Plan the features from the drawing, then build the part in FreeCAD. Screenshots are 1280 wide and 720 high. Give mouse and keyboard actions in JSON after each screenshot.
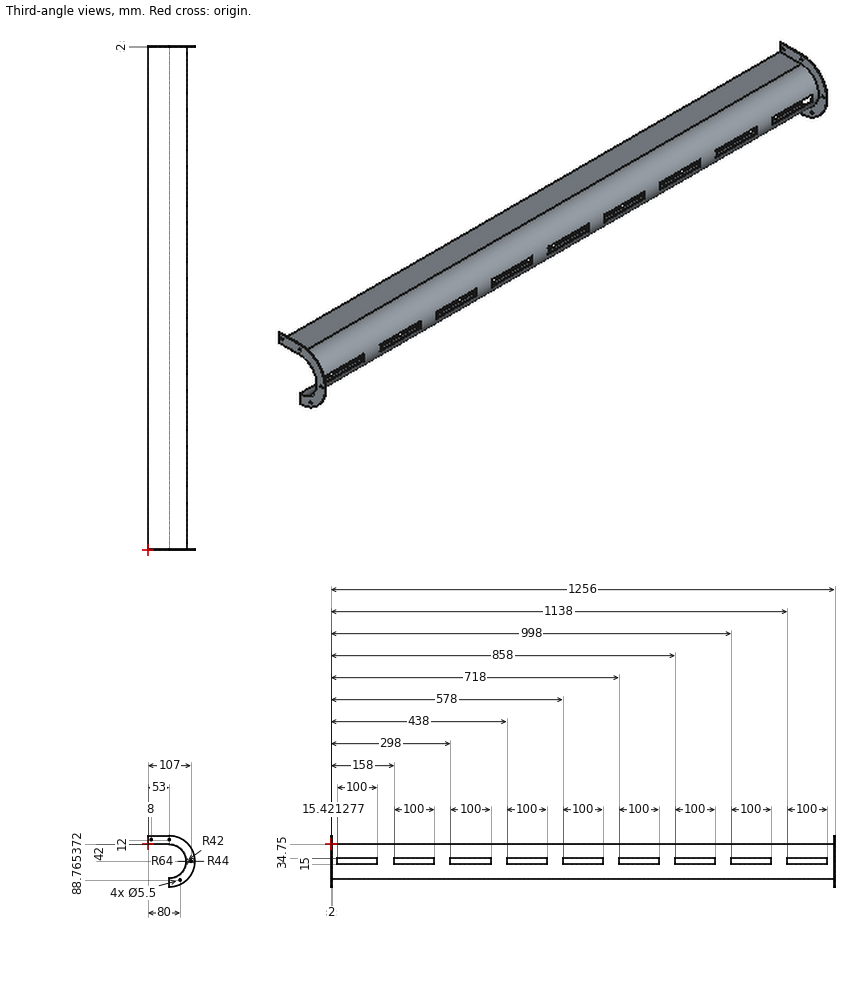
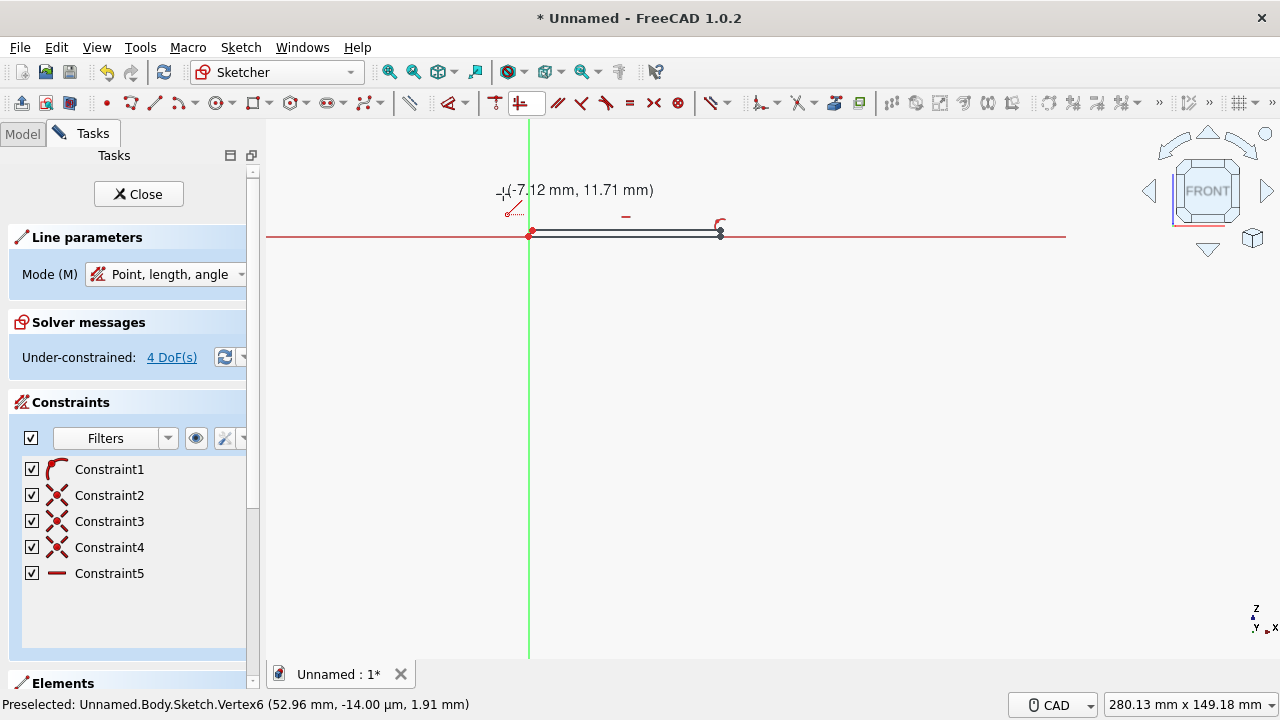
{"action": "left_click", "coordinate": [721, 548]}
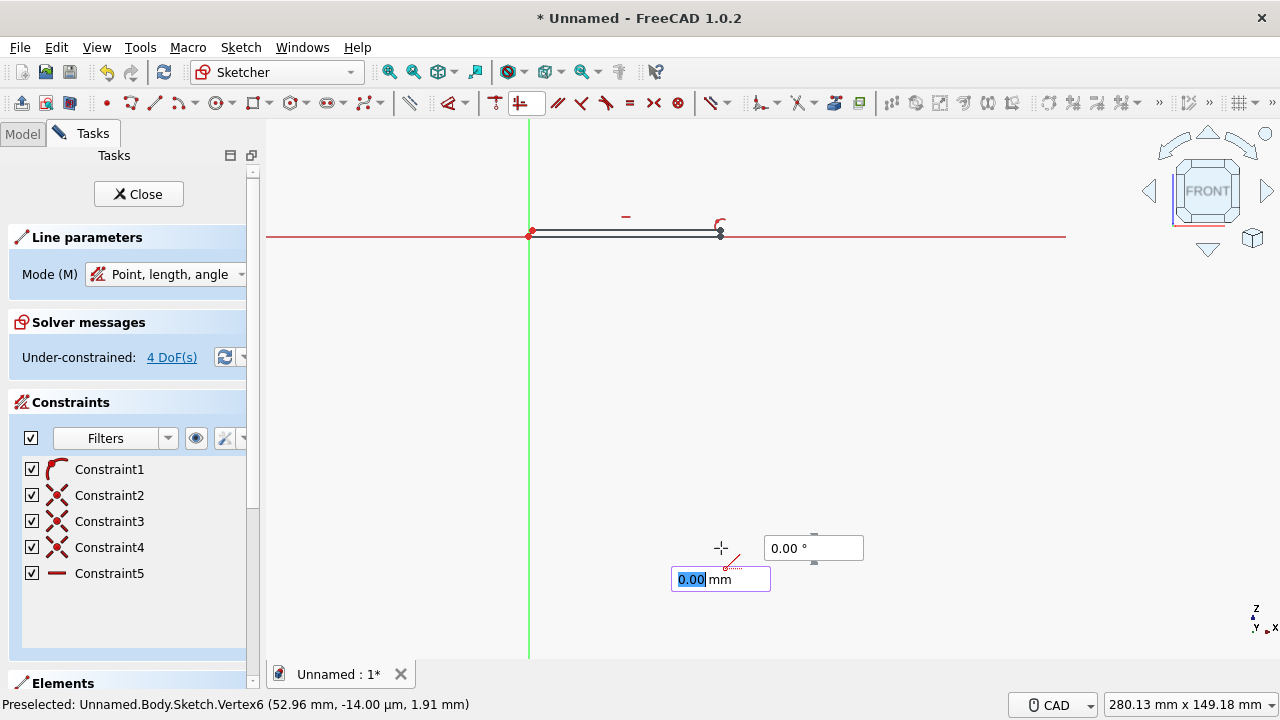
{"action": "scroll", "coordinate": [721, 541], "scroll_direction": "up", "scroll_amount": 4}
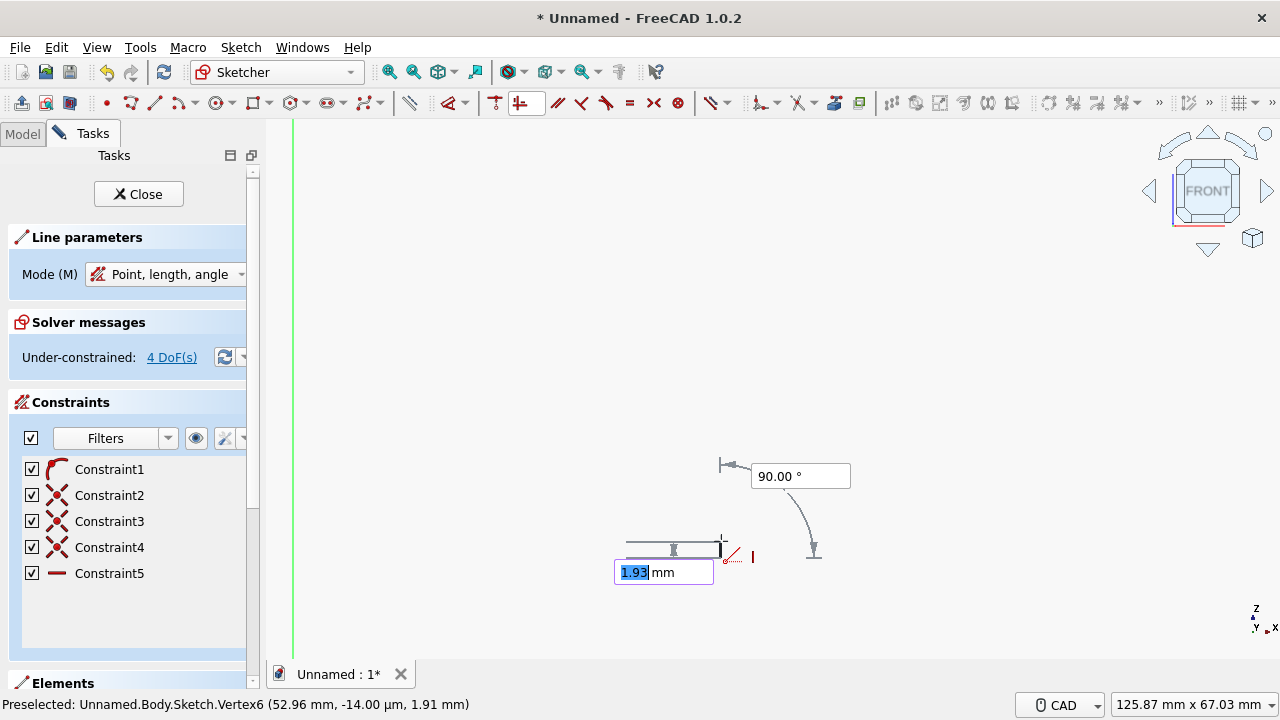
{"action": "left_click", "coordinate": [720, 540]}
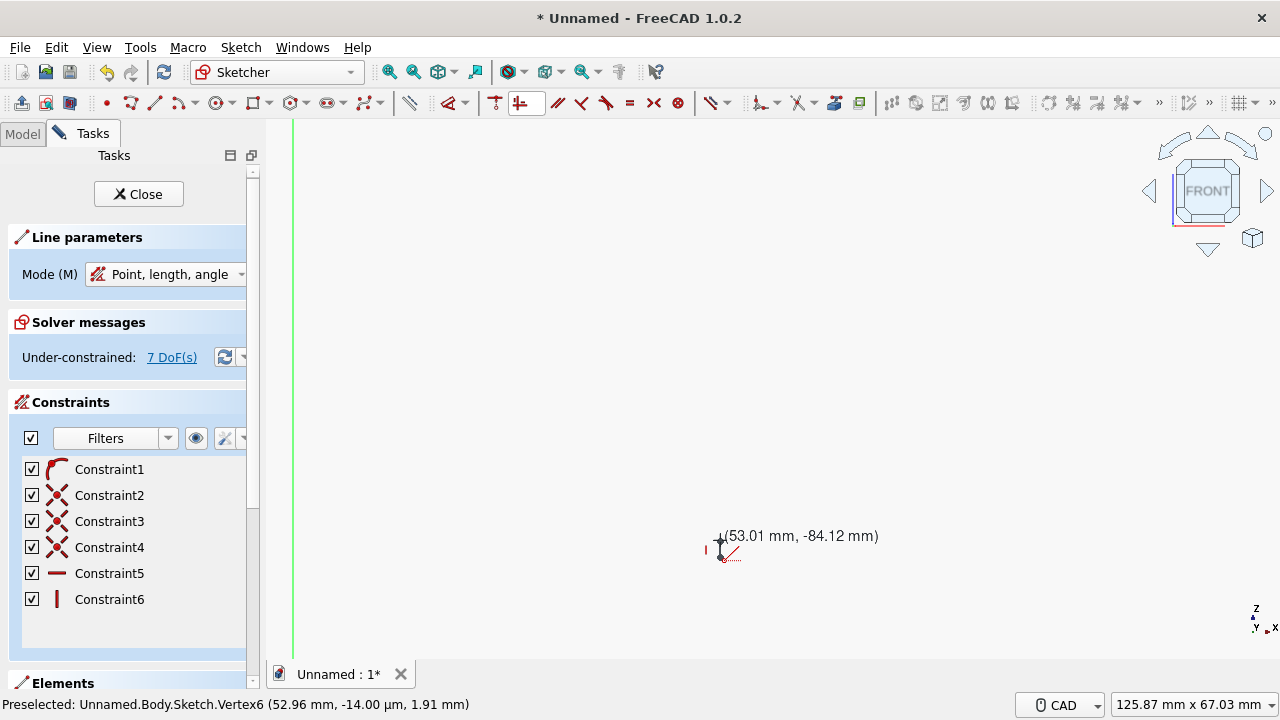
{"action": "left_click", "coordinate": [198, 104]}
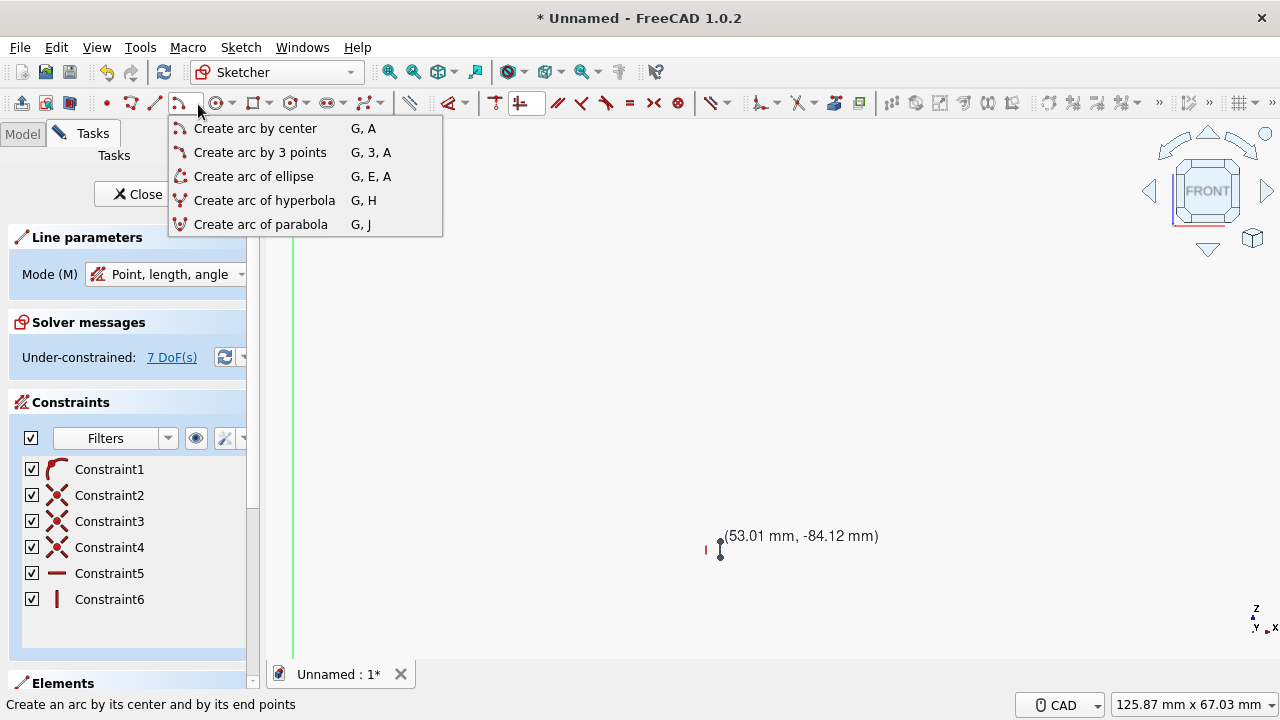
{"action": "left_click", "coordinate": [306, 152]}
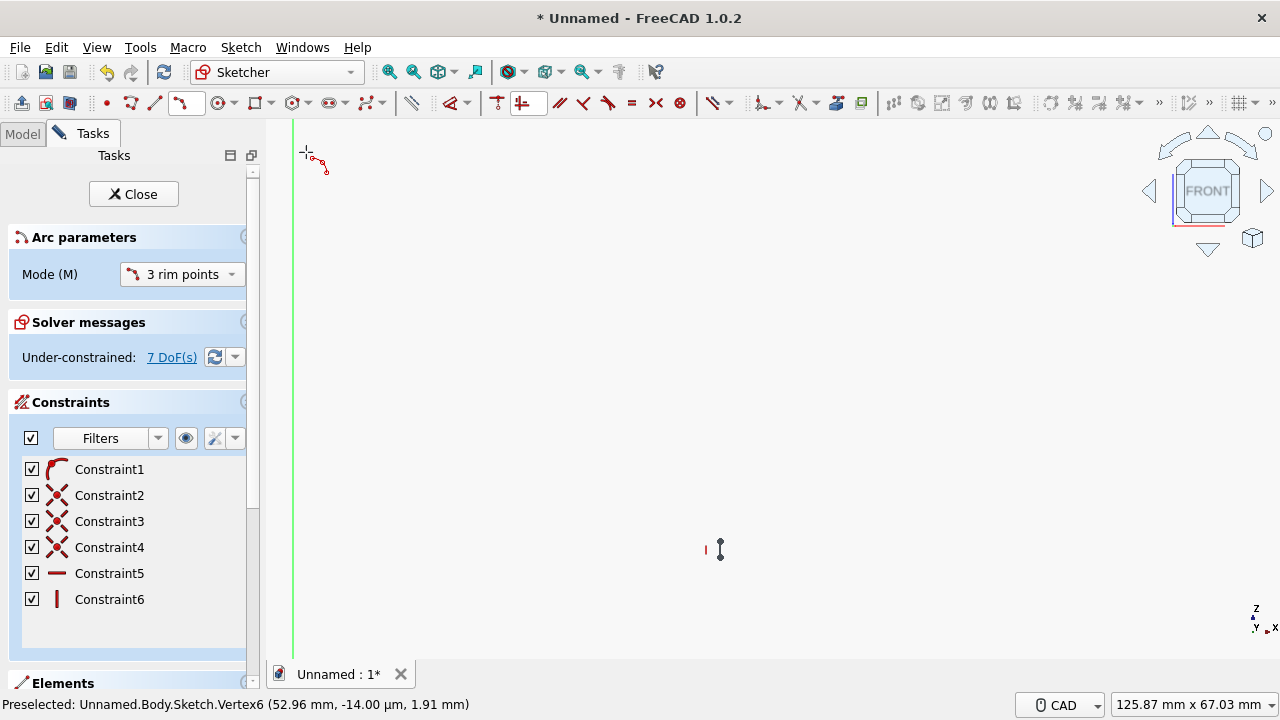
{"action": "scroll", "coordinate": [722, 542], "scroll_direction": "down", "scroll_amount": 4}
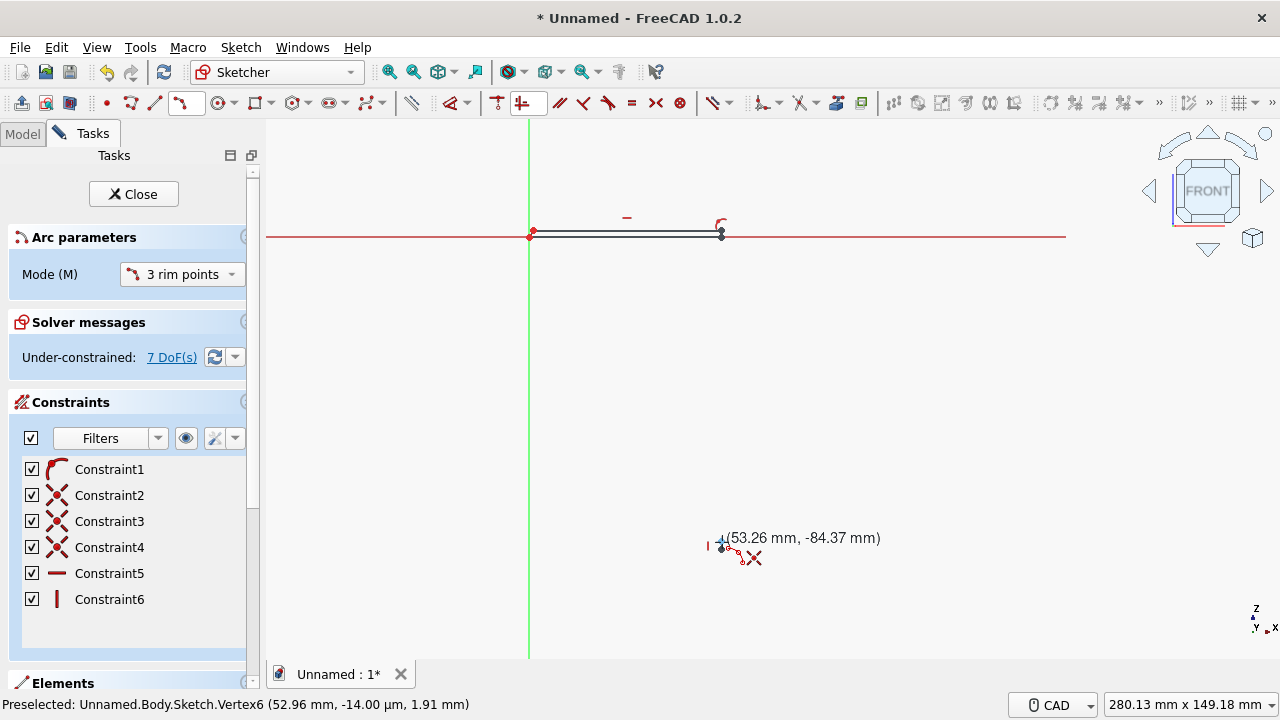
{"action": "scroll", "coordinate": [721, 230], "scroll_direction": "up", "scroll_amount": 4}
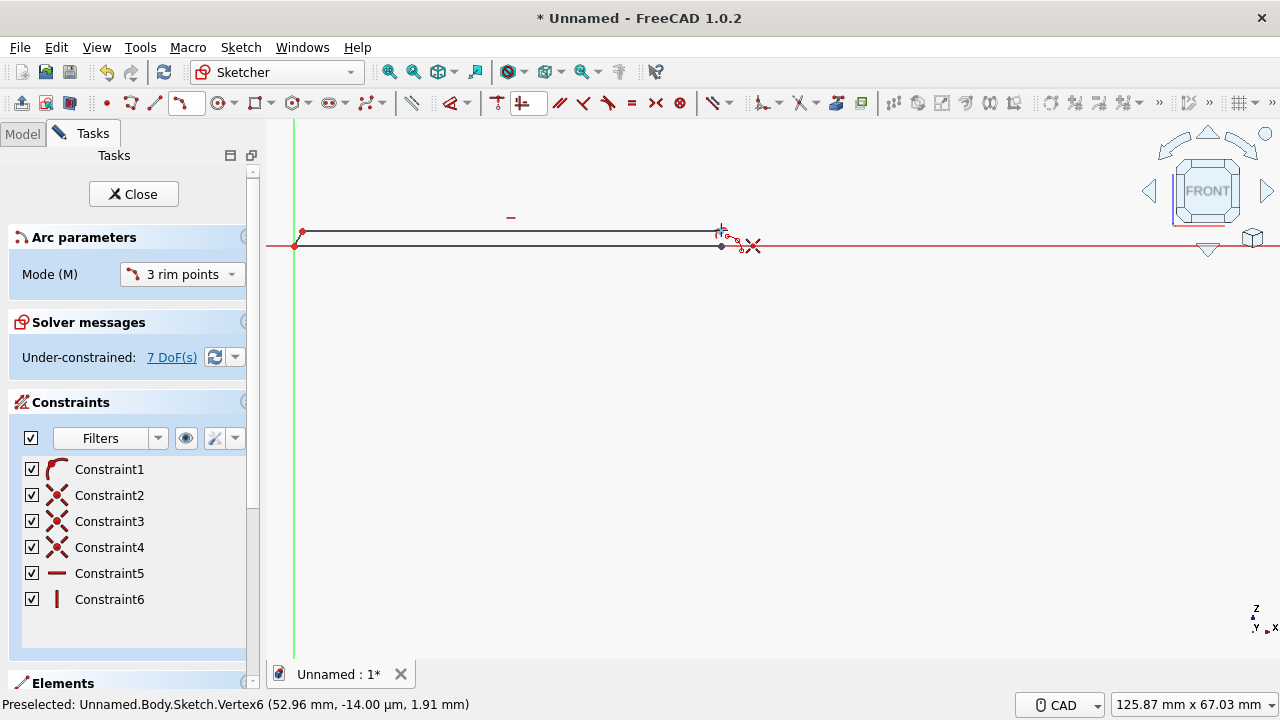
{"action": "left_click", "coordinate": [721, 231]}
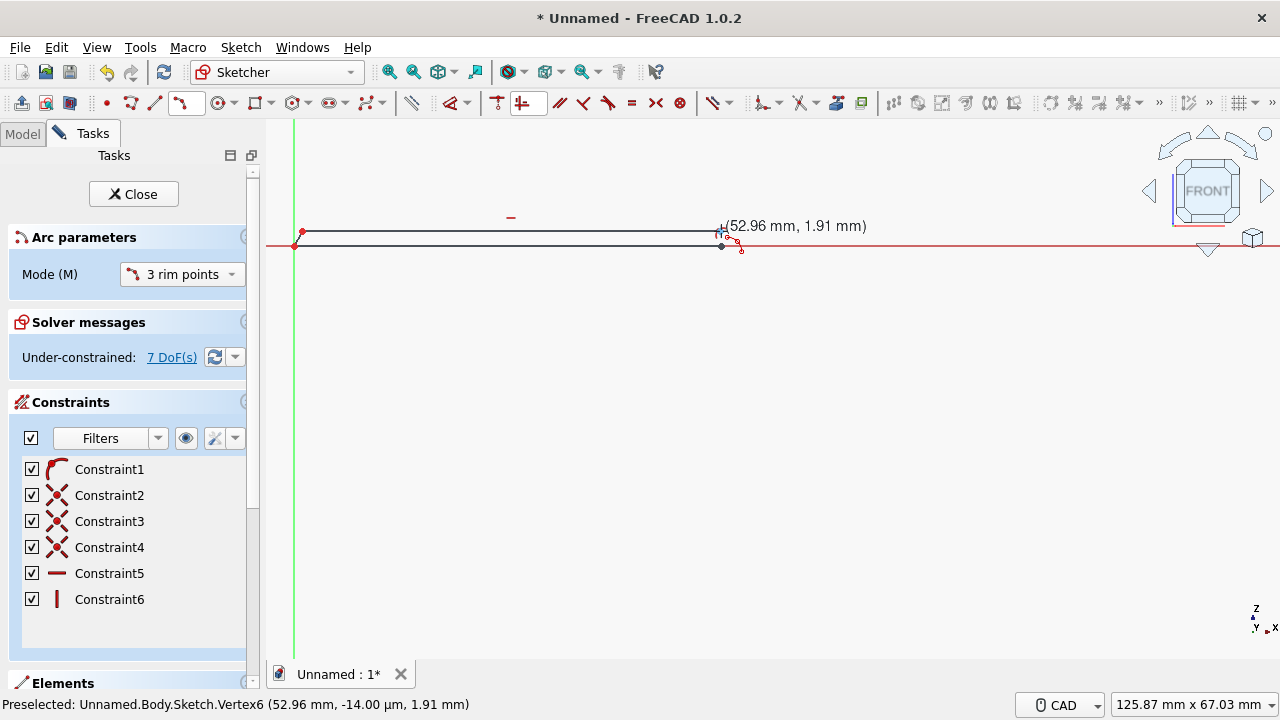
{"action": "scroll", "coordinate": [721, 229], "scroll_direction": "down", "scroll_amount": 4}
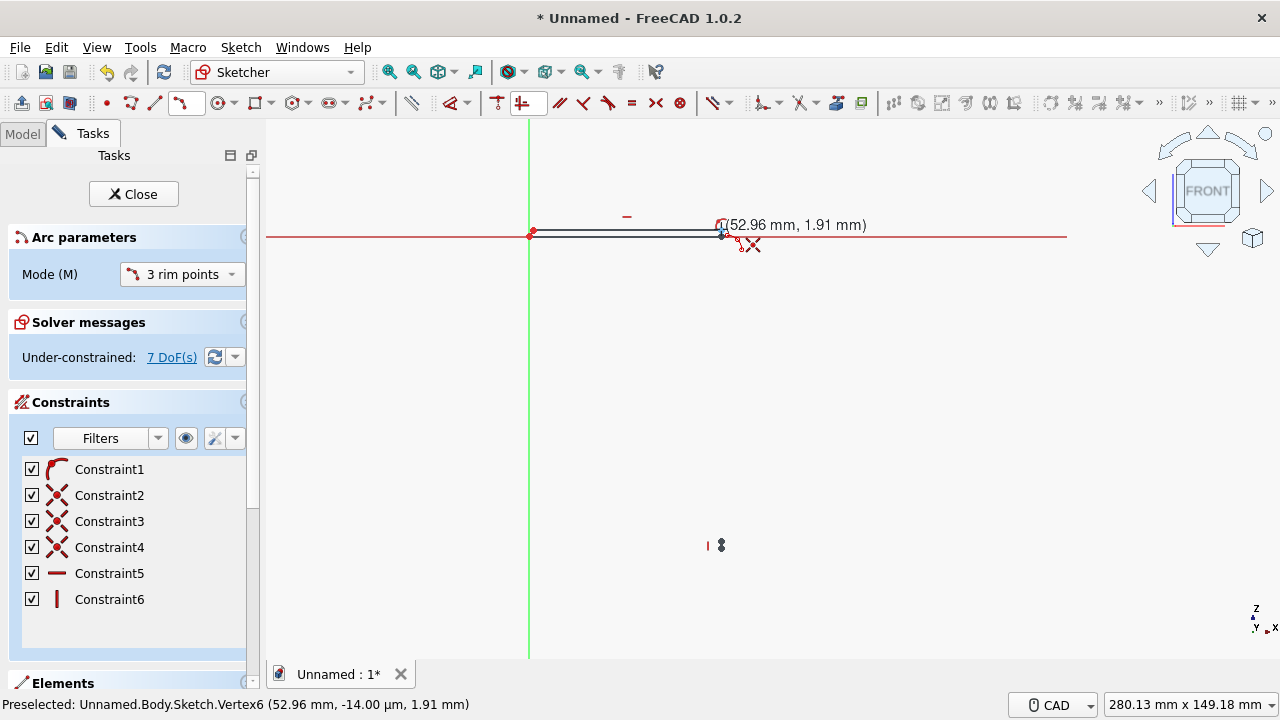
{"action": "scroll", "coordinate": [721, 548], "scroll_direction": "up", "scroll_amount": 8}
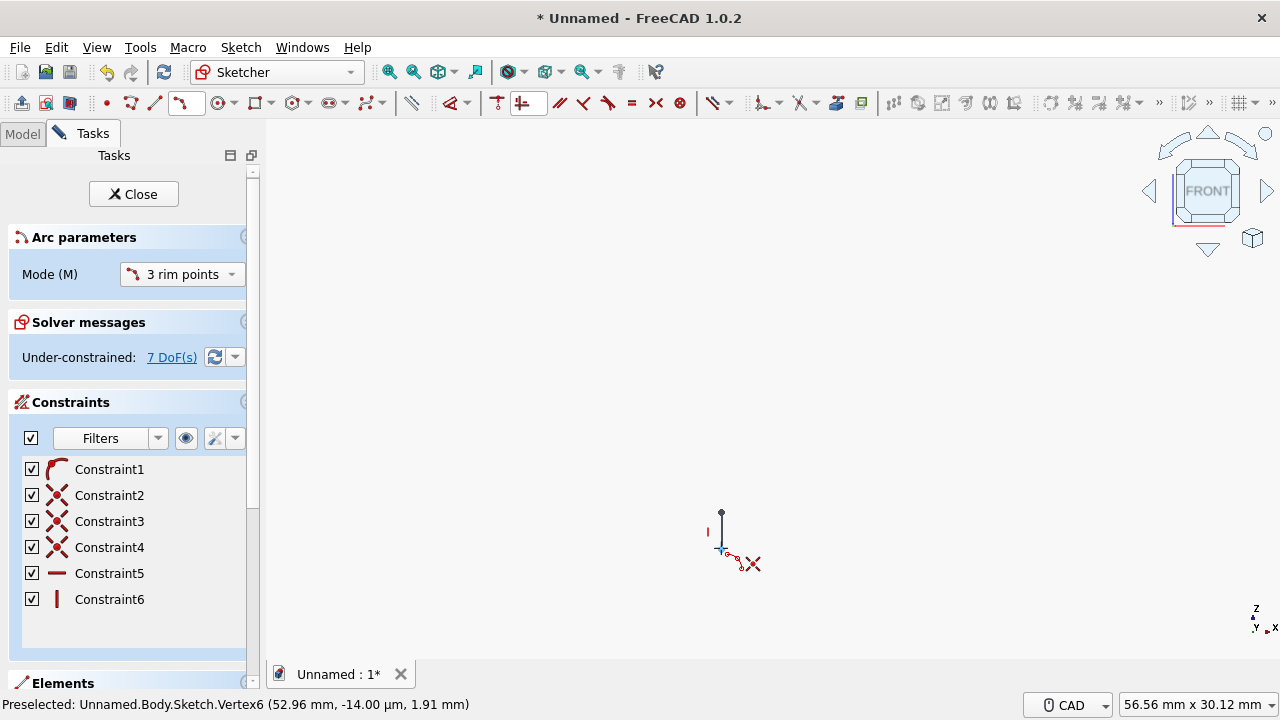
{"action": "left_click", "coordinate": [722, 550]}